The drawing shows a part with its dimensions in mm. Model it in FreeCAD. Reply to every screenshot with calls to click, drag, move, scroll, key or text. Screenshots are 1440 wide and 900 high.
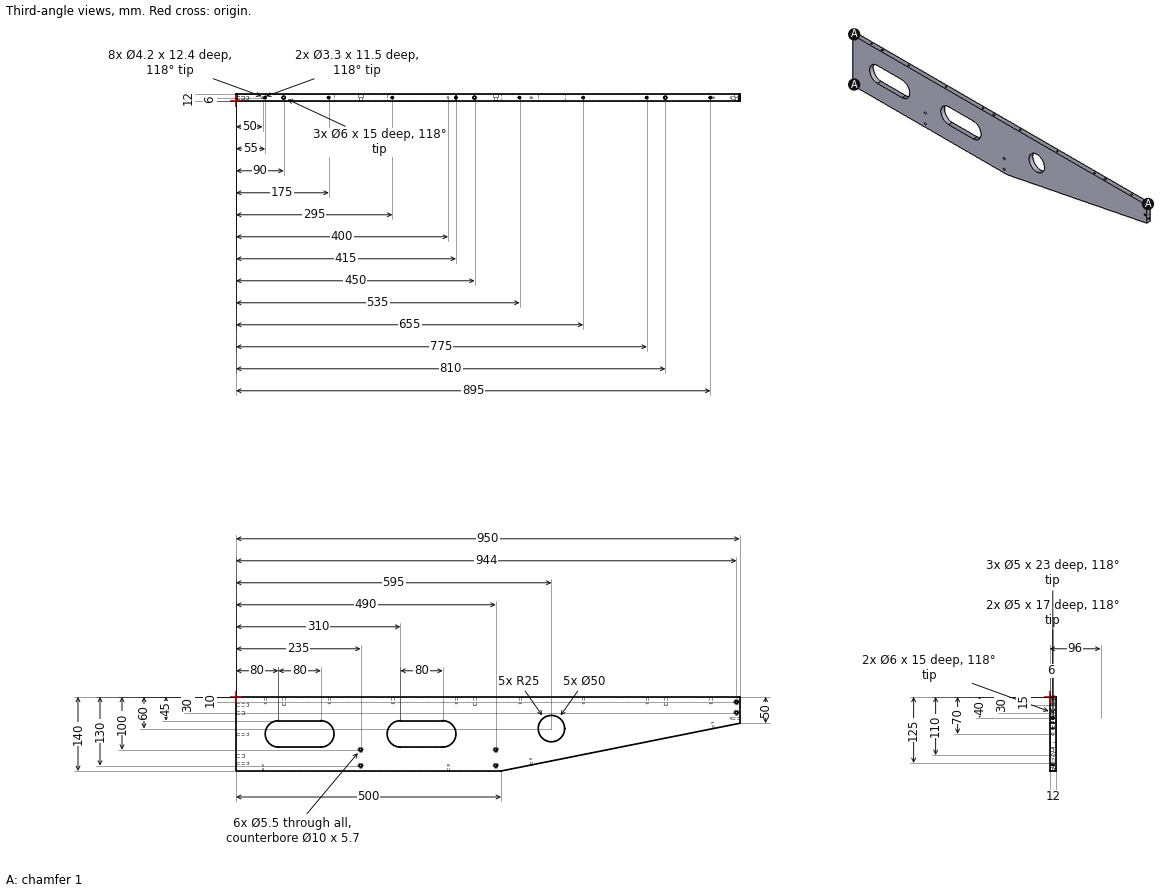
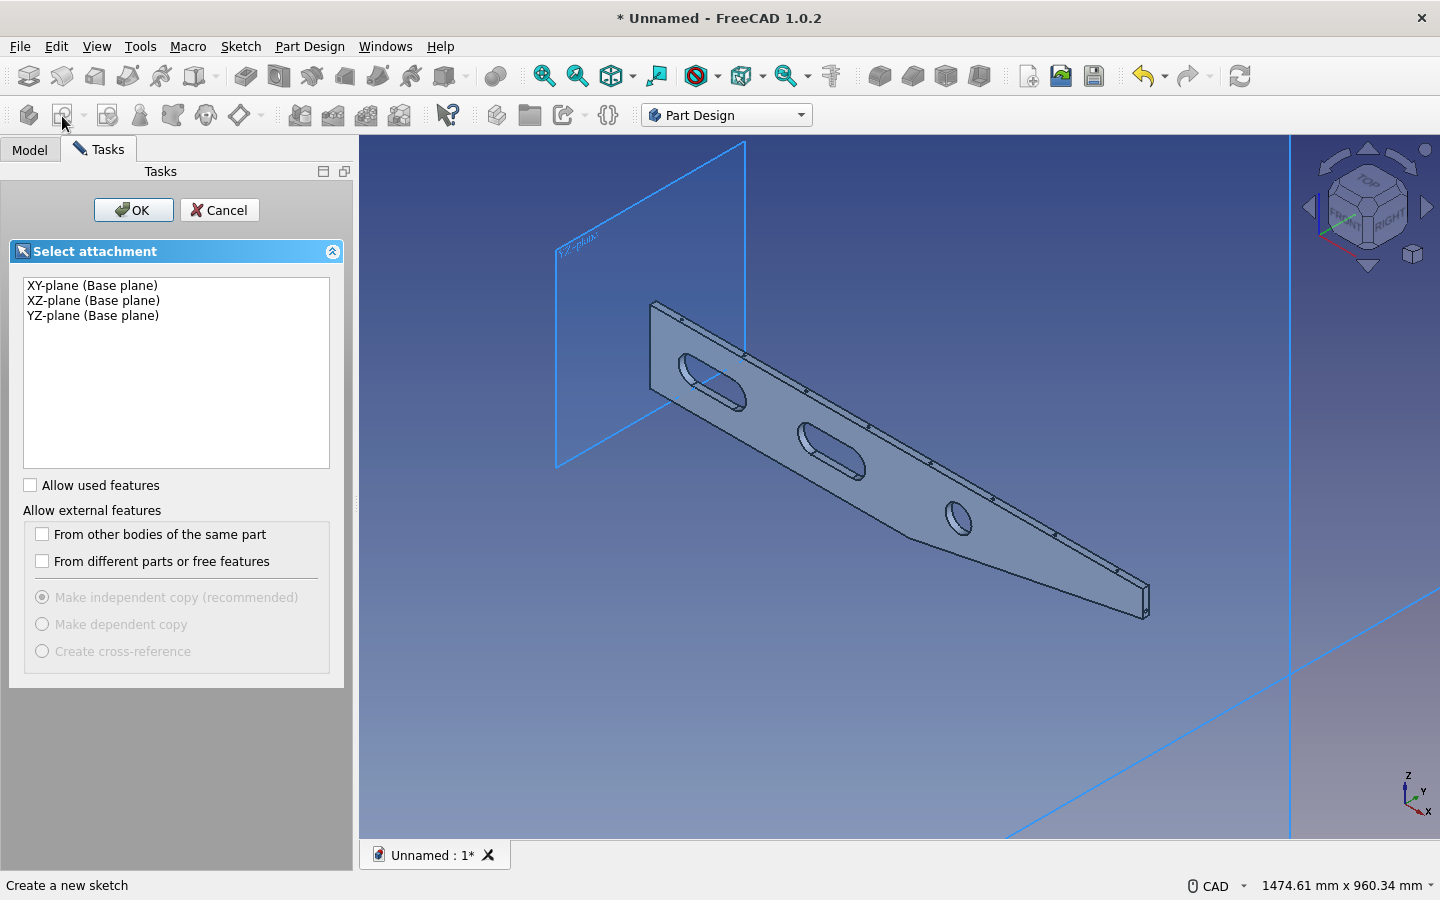
click(84, 286)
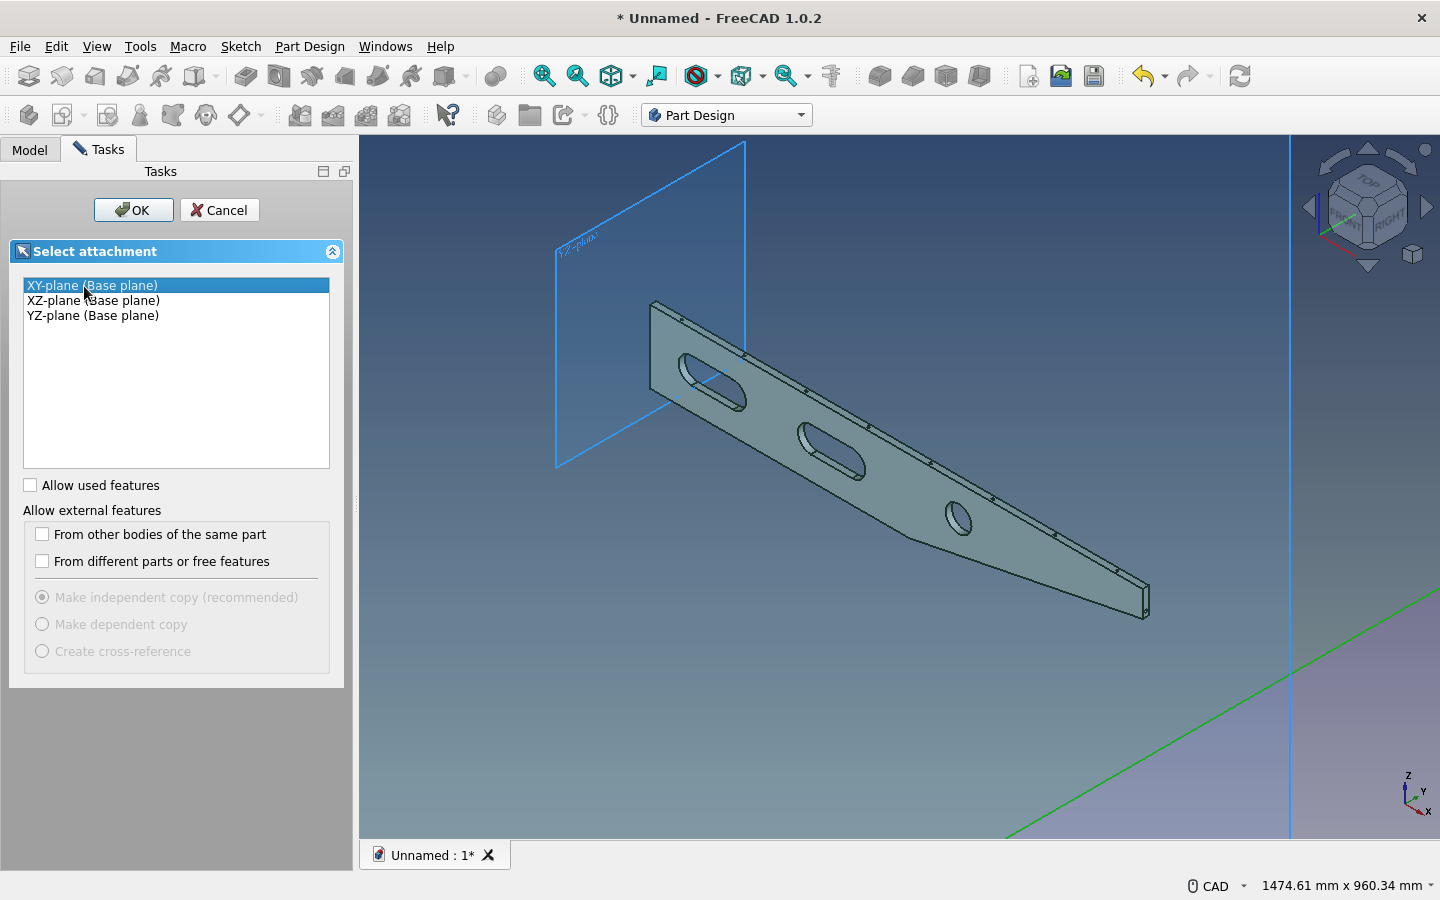
click(134, 210)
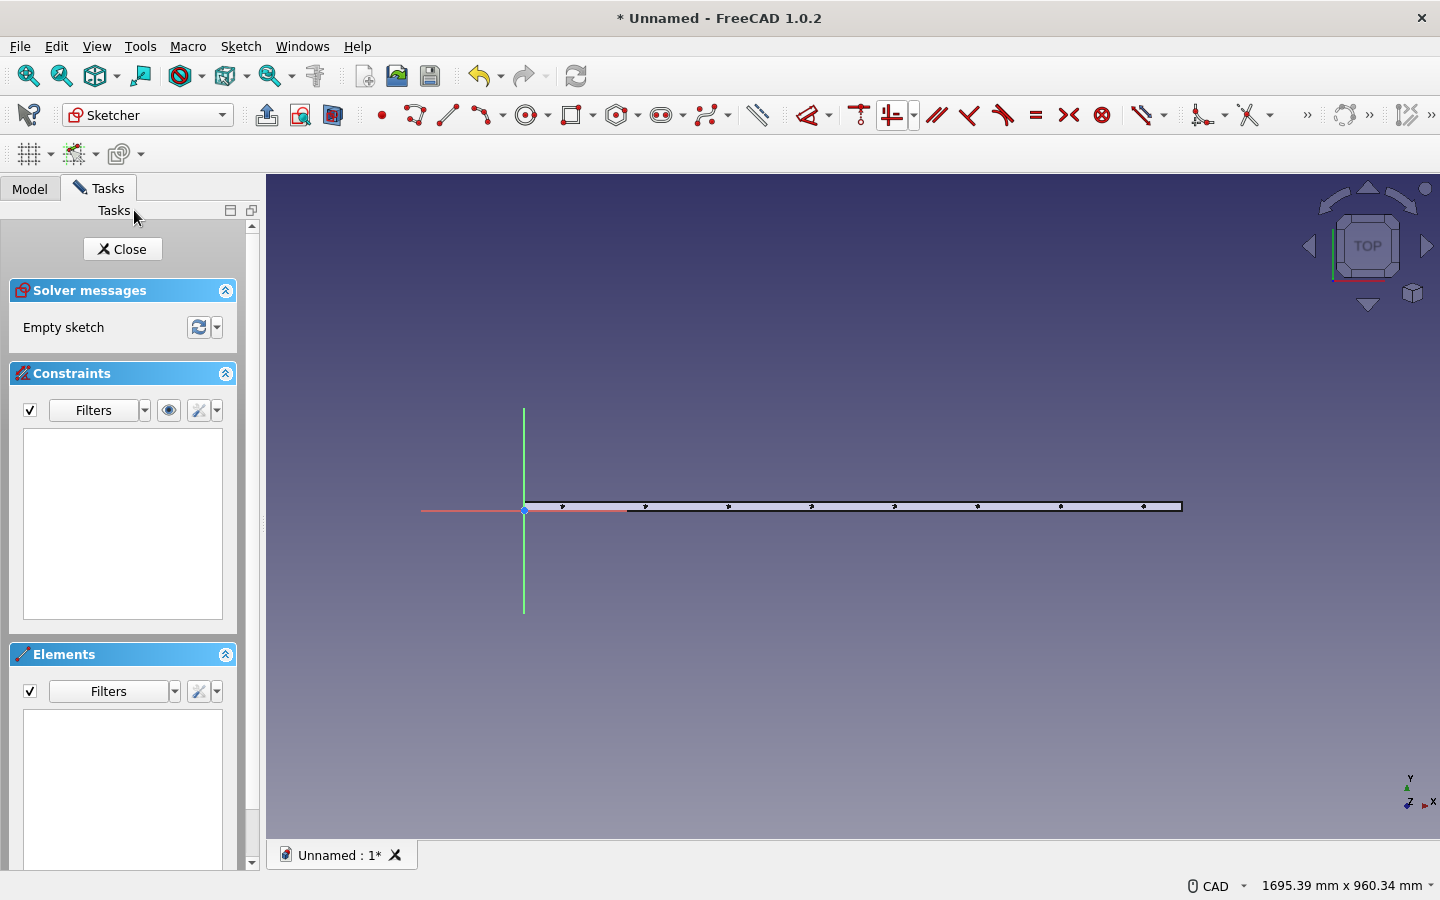
click(526, 116)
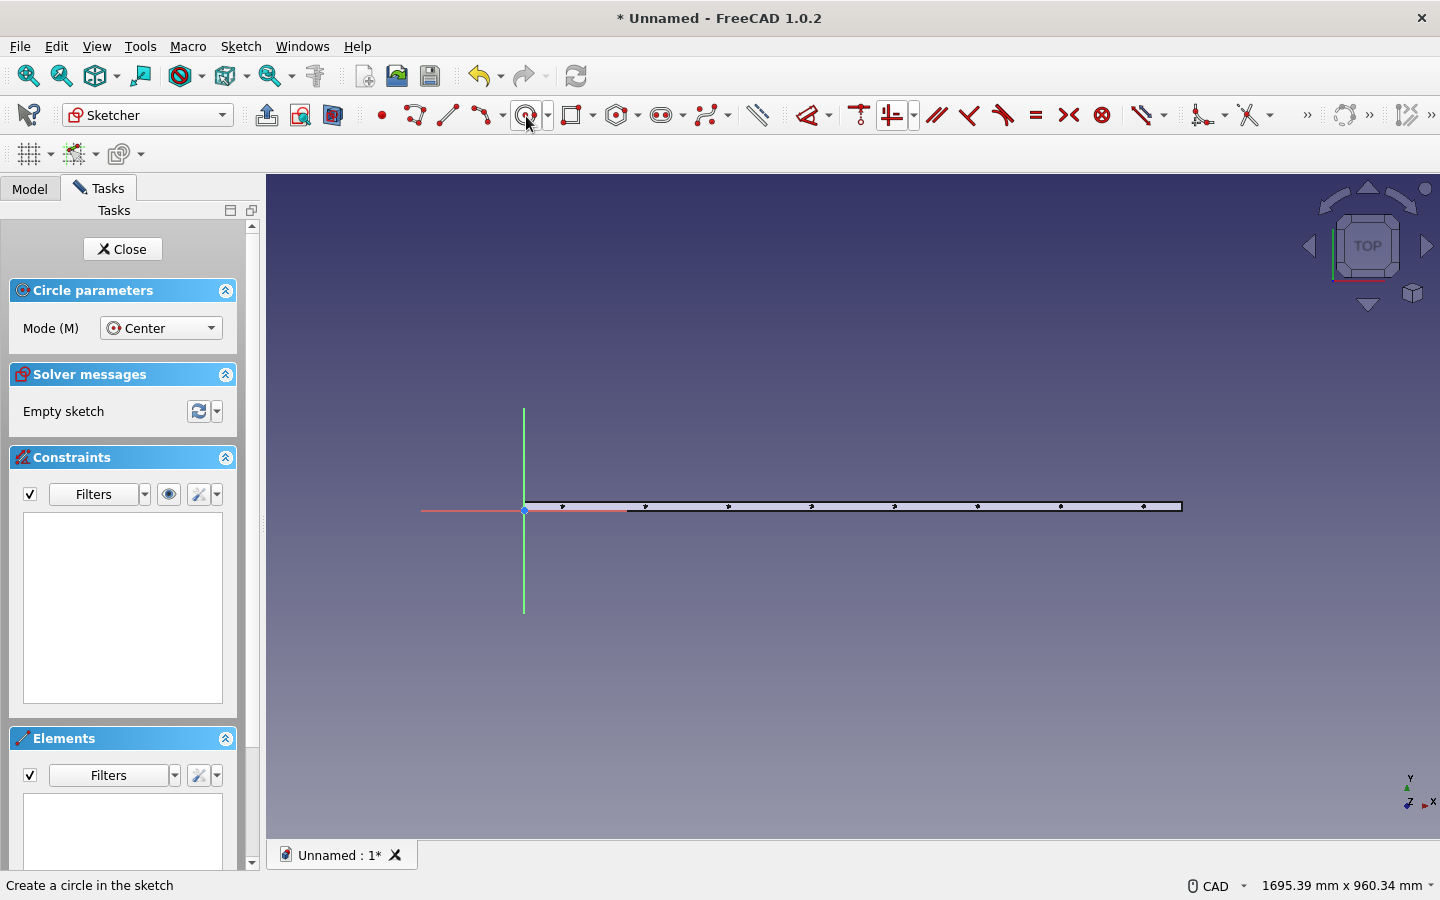
scroll(586, 506, up, 12)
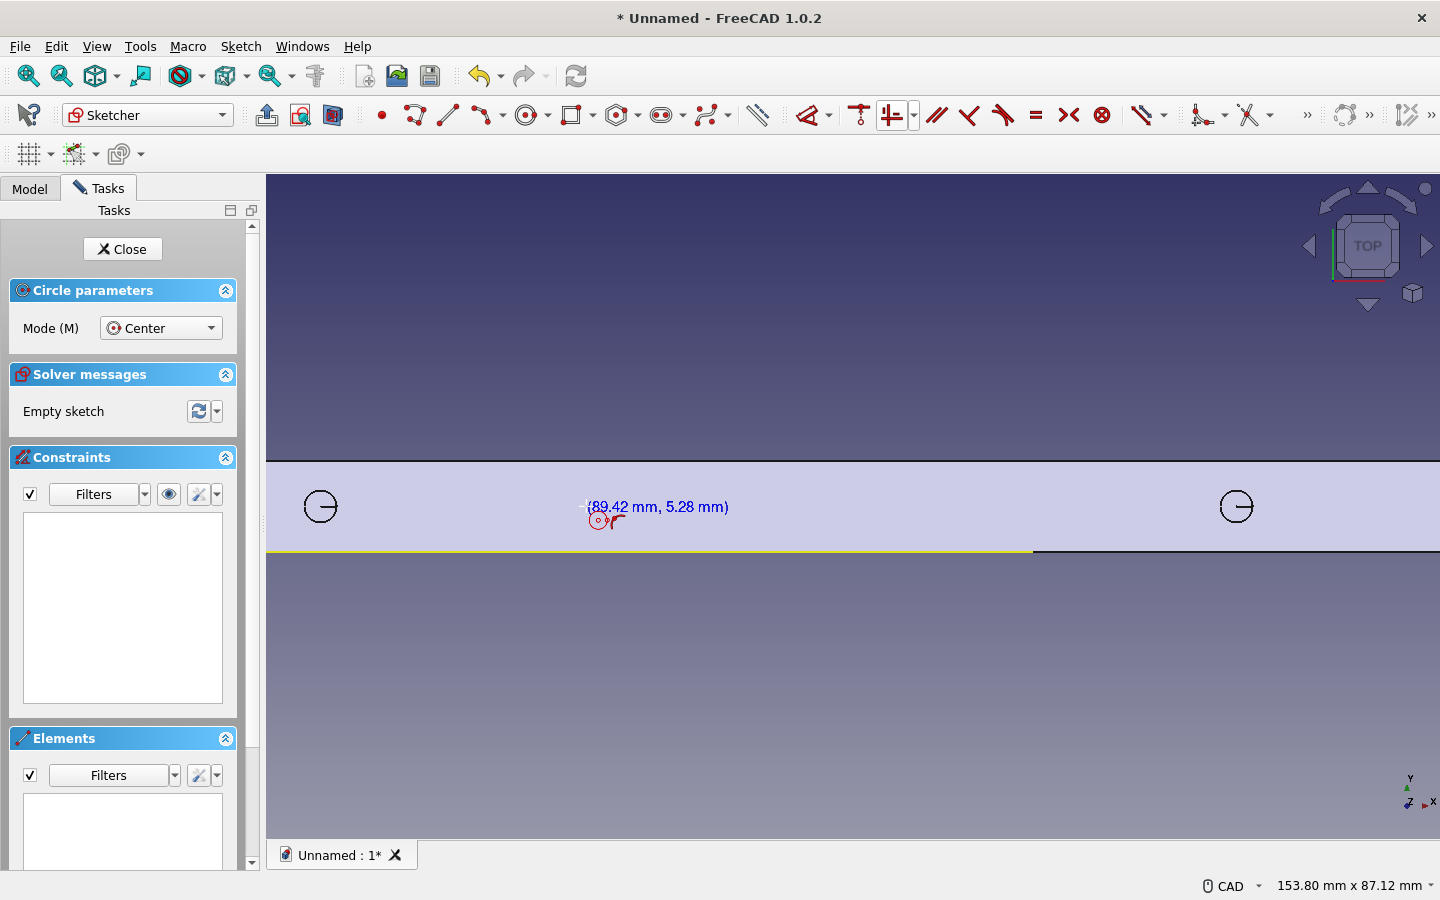
scroll(508, 505, down, 11)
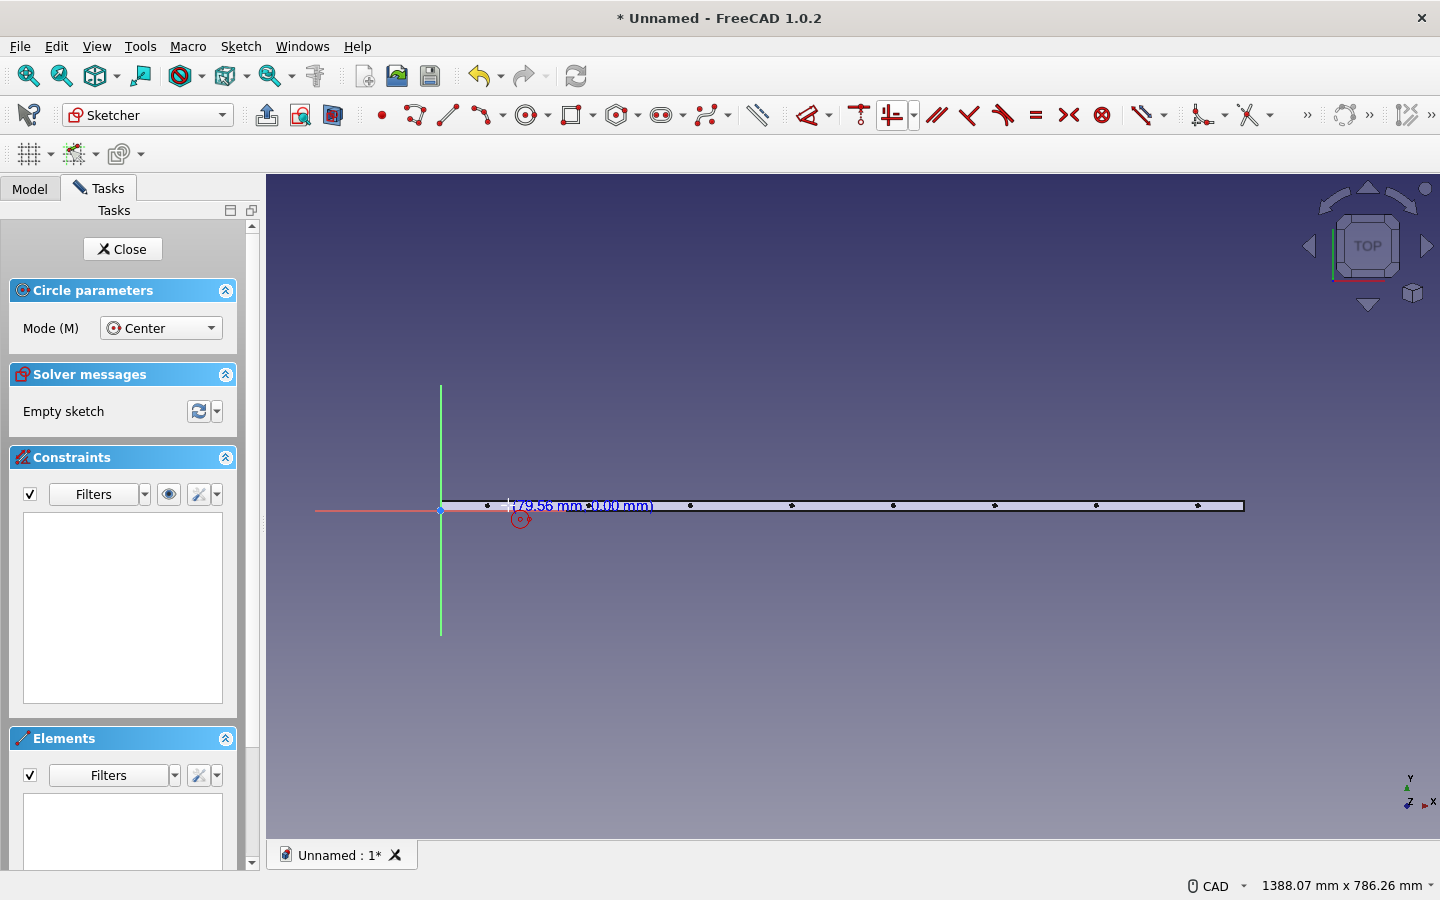
scroll(517, 506, up, 6)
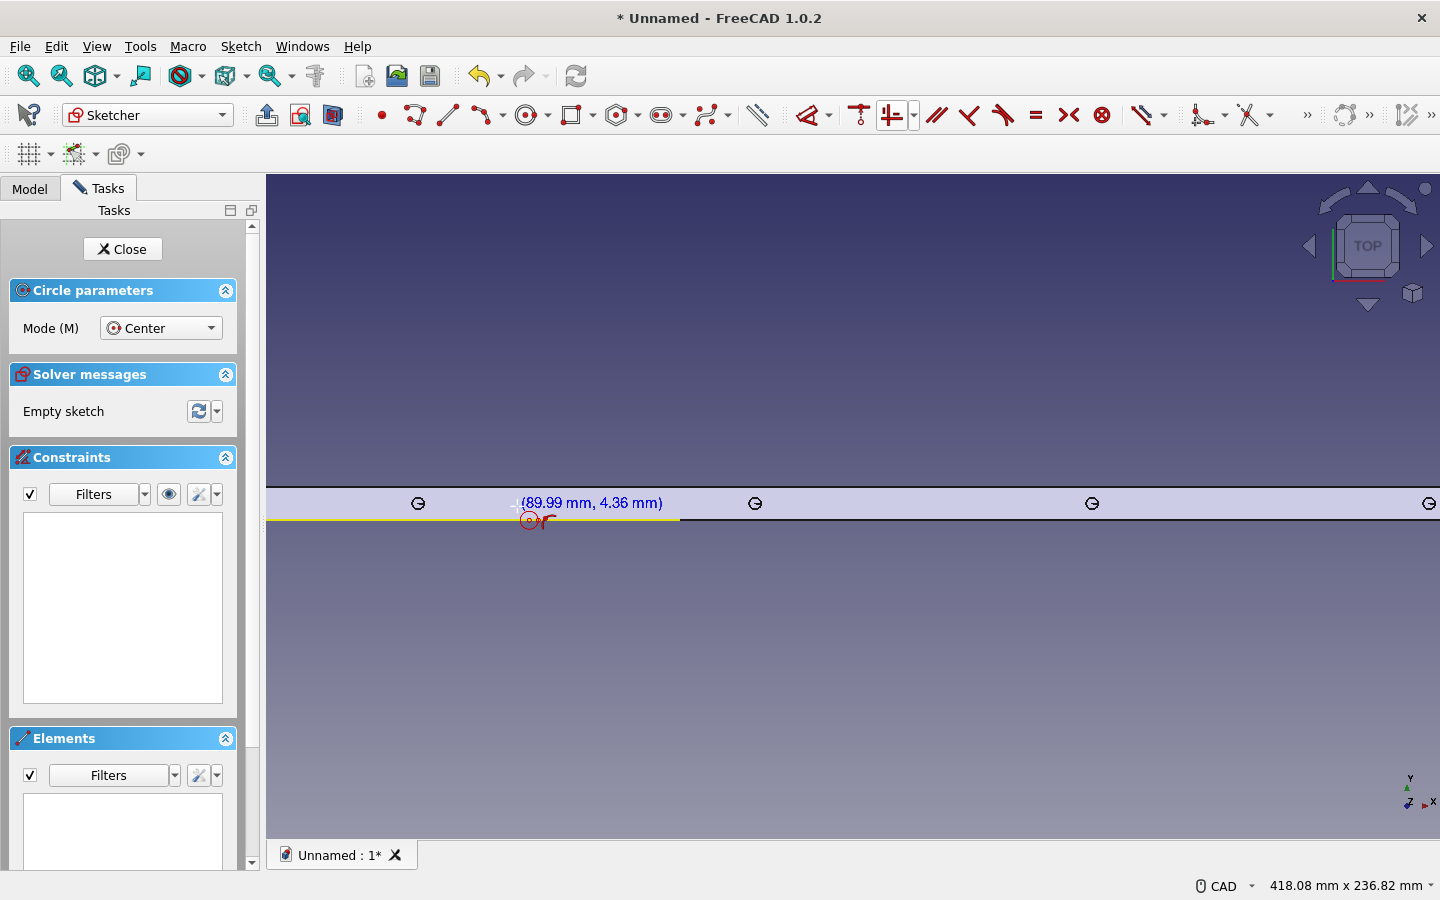
click(517, 504)
move(523, 498)